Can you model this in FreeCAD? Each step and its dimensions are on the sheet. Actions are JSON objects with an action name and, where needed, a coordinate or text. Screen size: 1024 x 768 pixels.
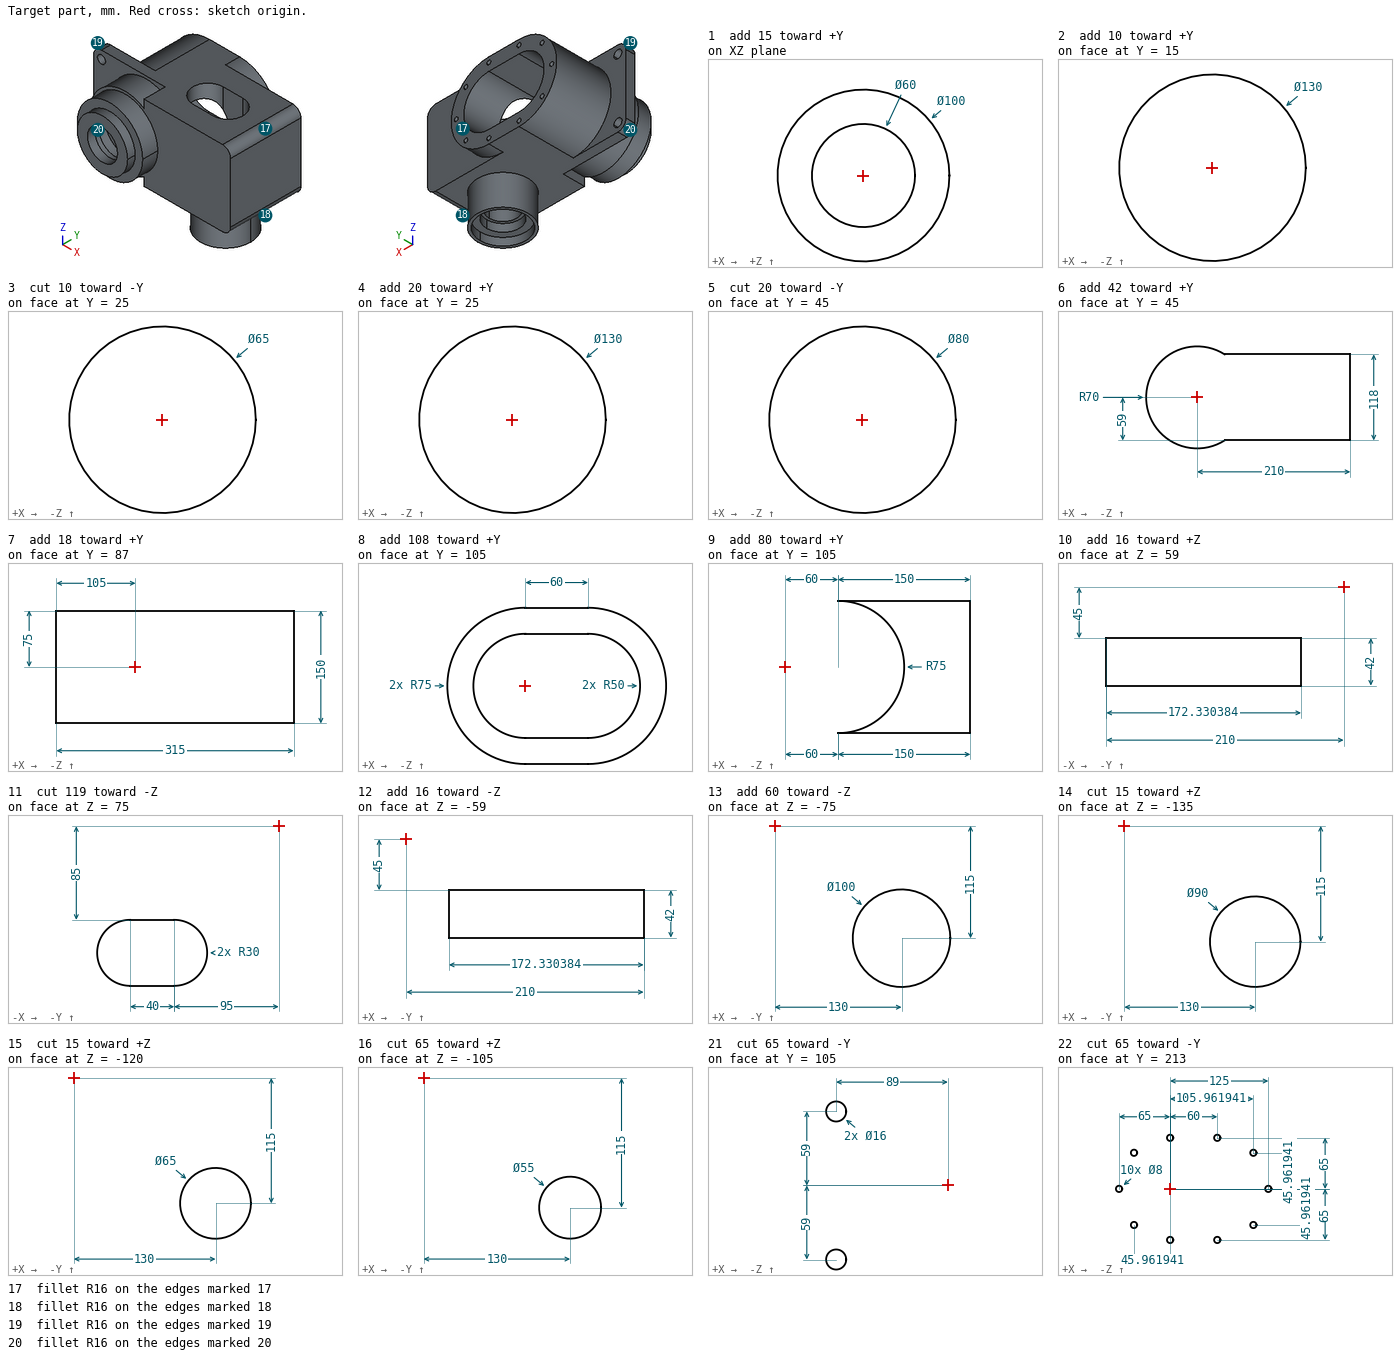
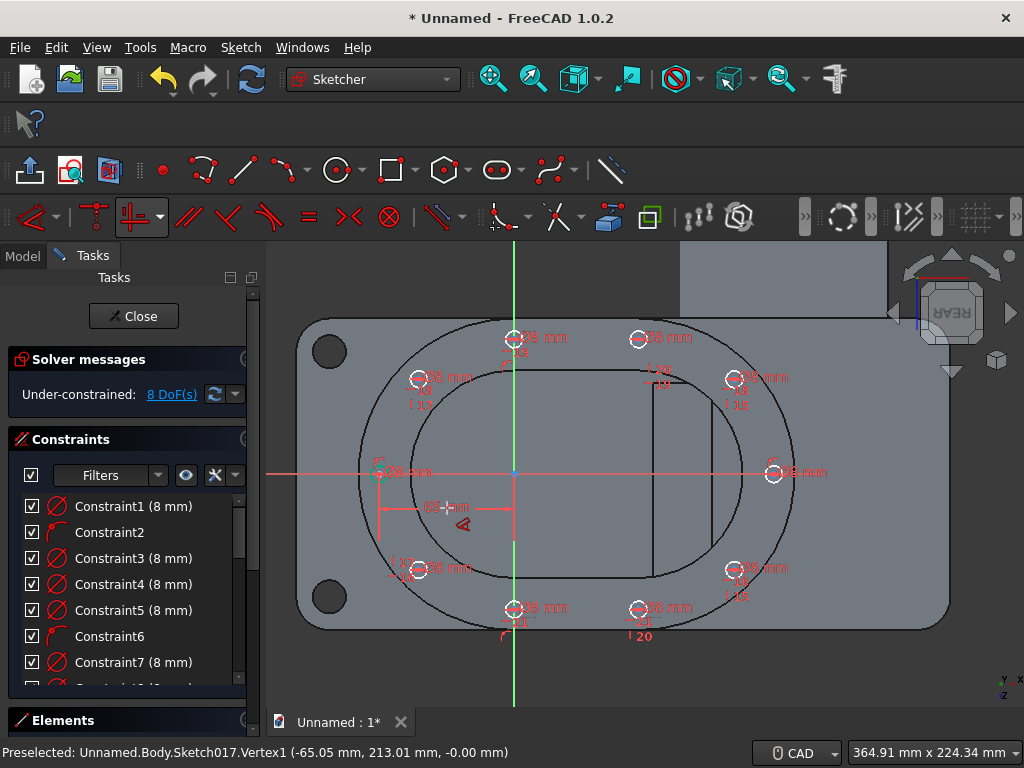
{"action": "left_click", "coordinate": [639, 339]}
{"action": "left_click", "coordinate": [576, 305]}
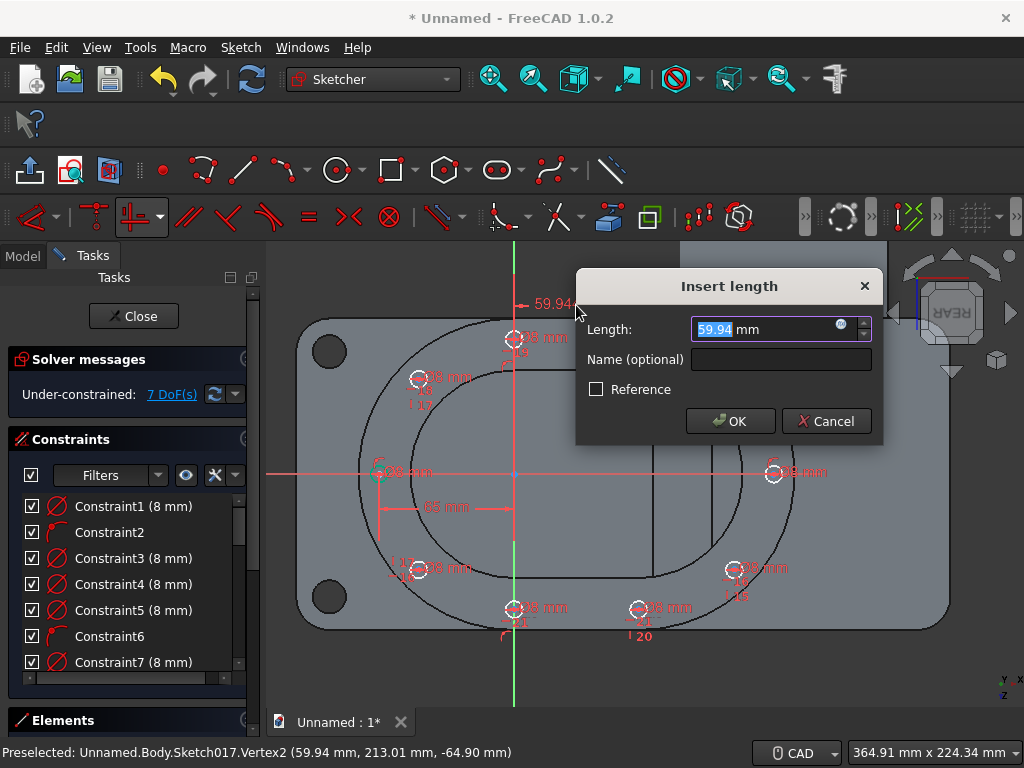
{"action": "type", "text": "60"}
{"action": "key", "text": "Return"}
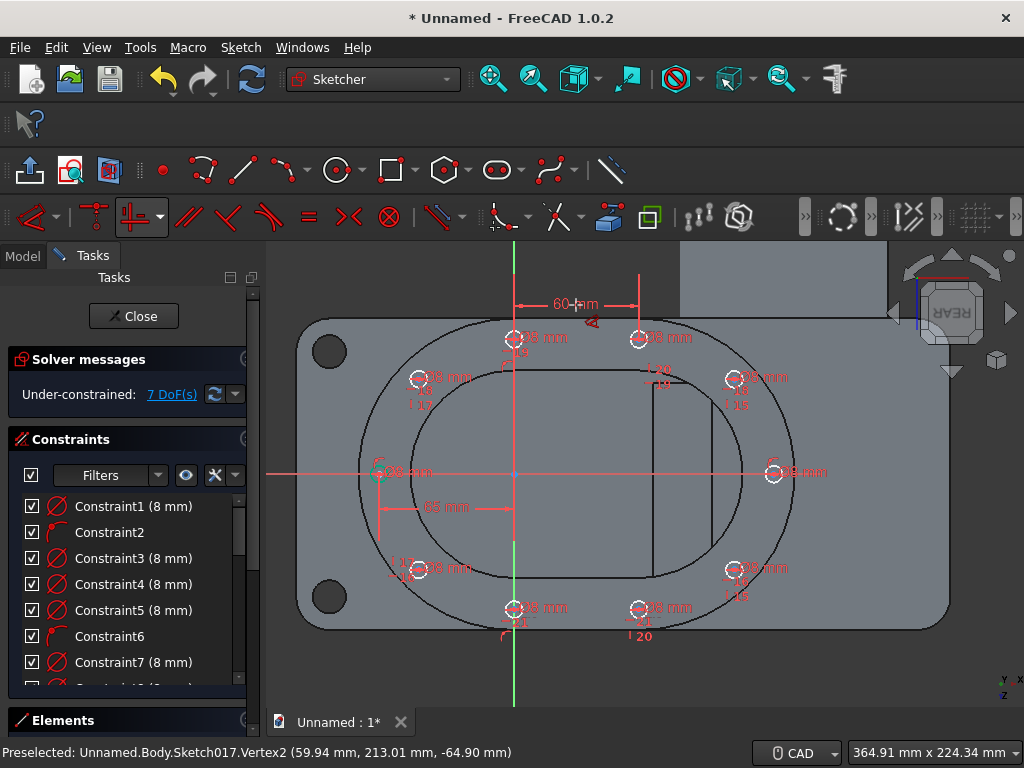
{"action": "left_click", "coordinate": [639, 339]}
{"action": "left_click", "coordinate": [673, 407]}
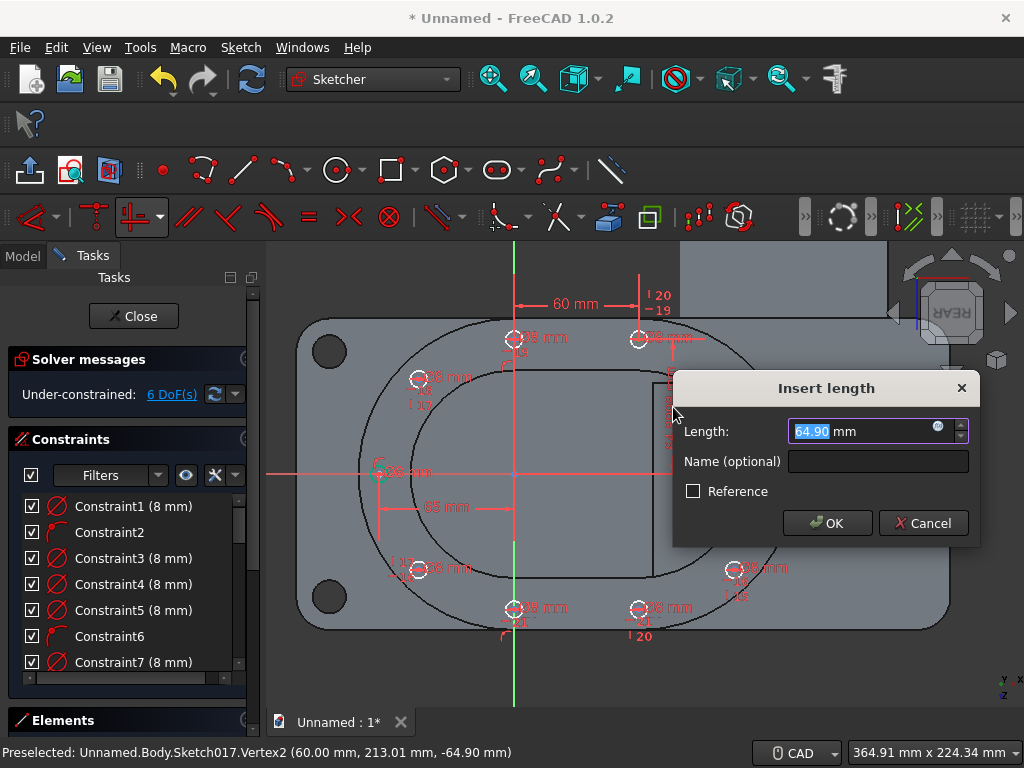
{"action": "type", "text": "65"}
{"action": "key", "text": "Return"}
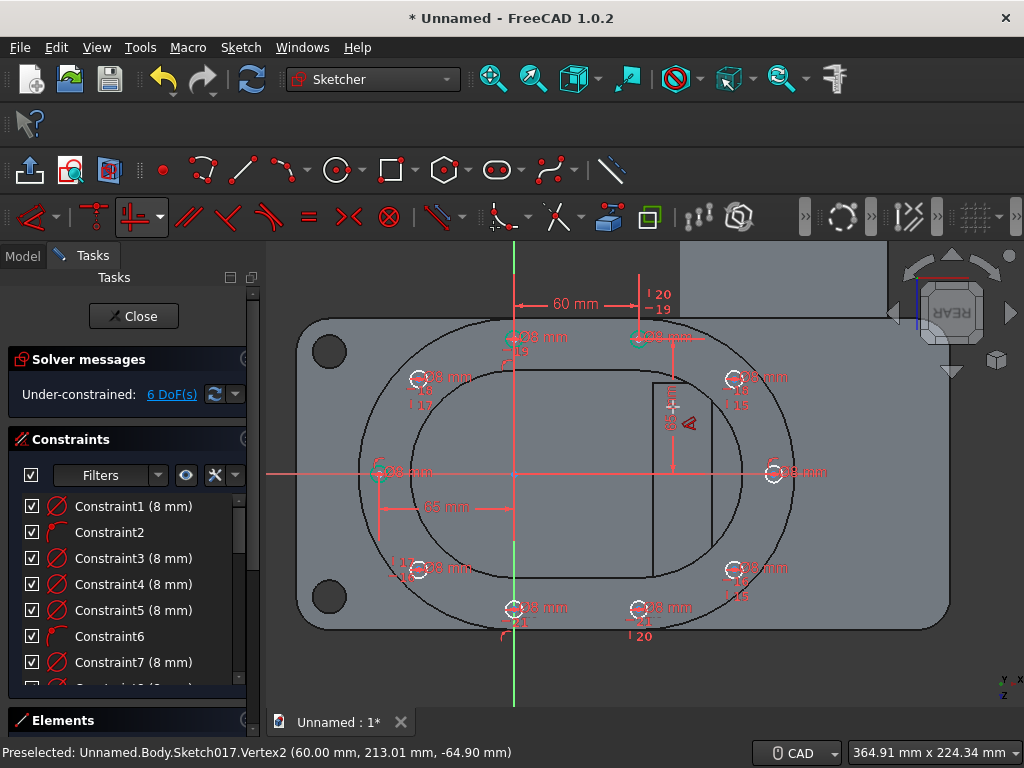
{"action": "left_click", "coordinate": [639, 610]}
{"action": "left_click", "coordinate": [673, 542]}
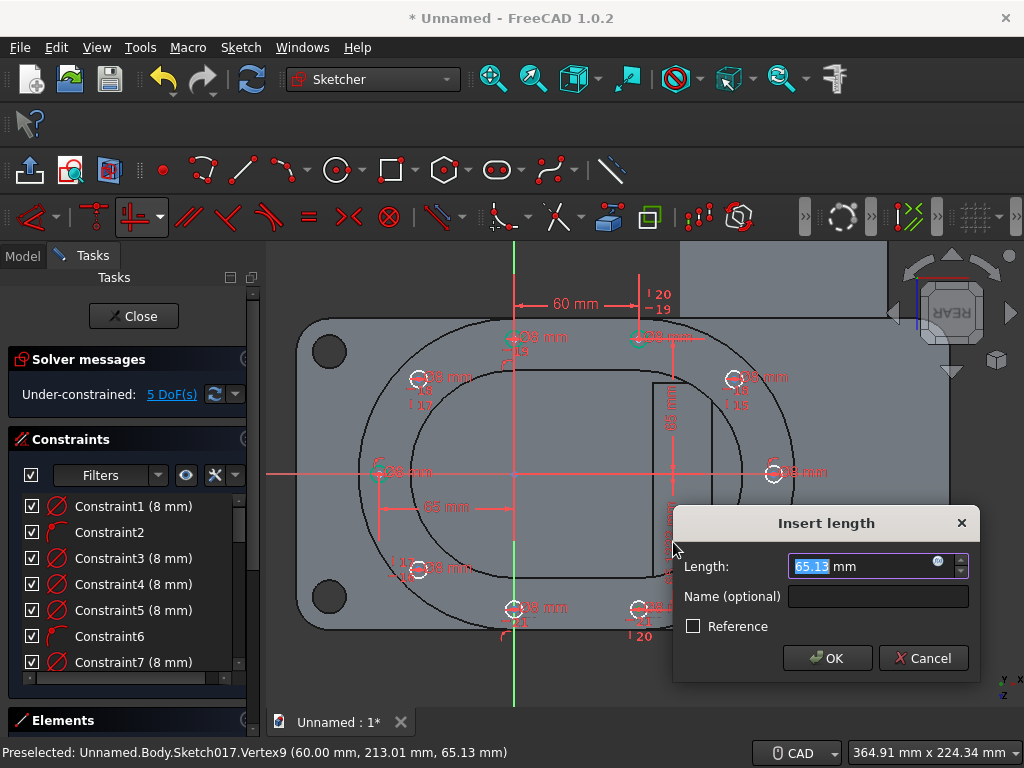
{"action": "type", "text": "65"}
{"action": "key", "text": "Return"}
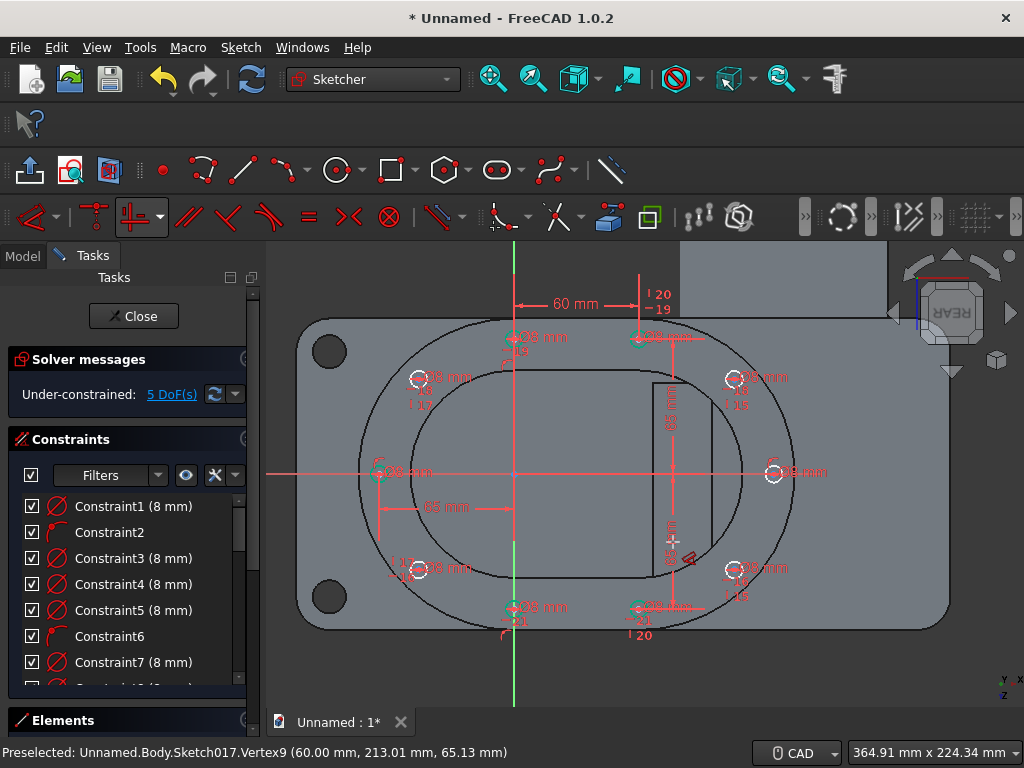
{"action": "left_click", "coordinate": [774, 474]}
{"action": "left_click", "coordinate": [644, 508]}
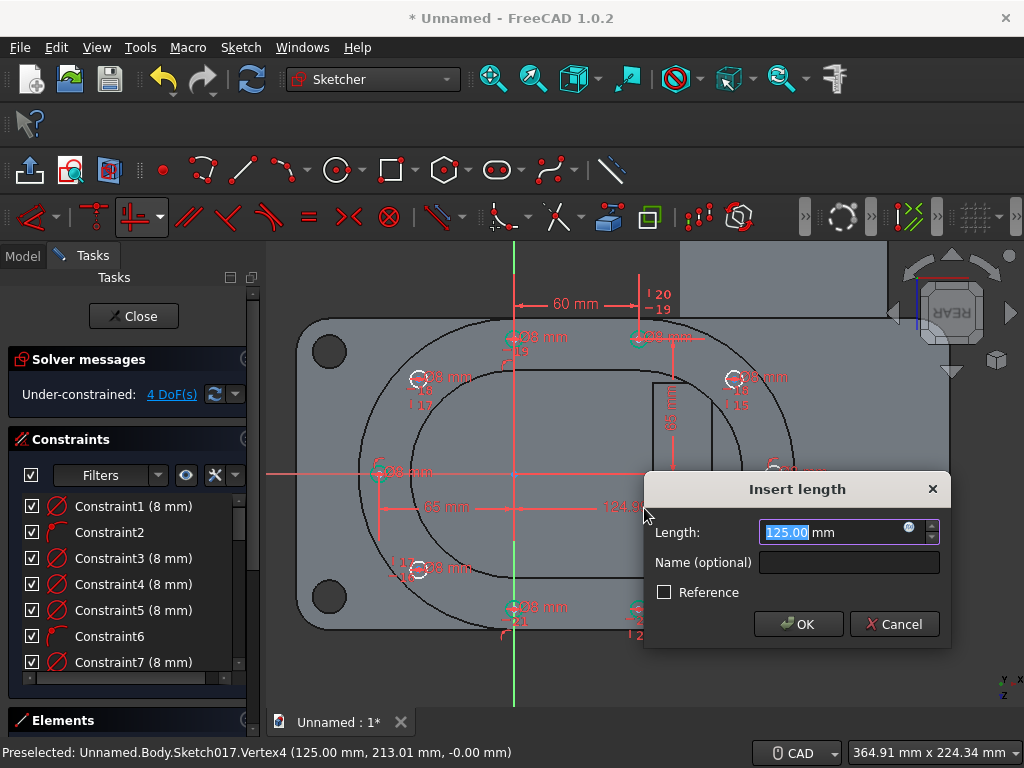
{"action": "type", "text": "125"}
{"action": "key", "text": "Return"}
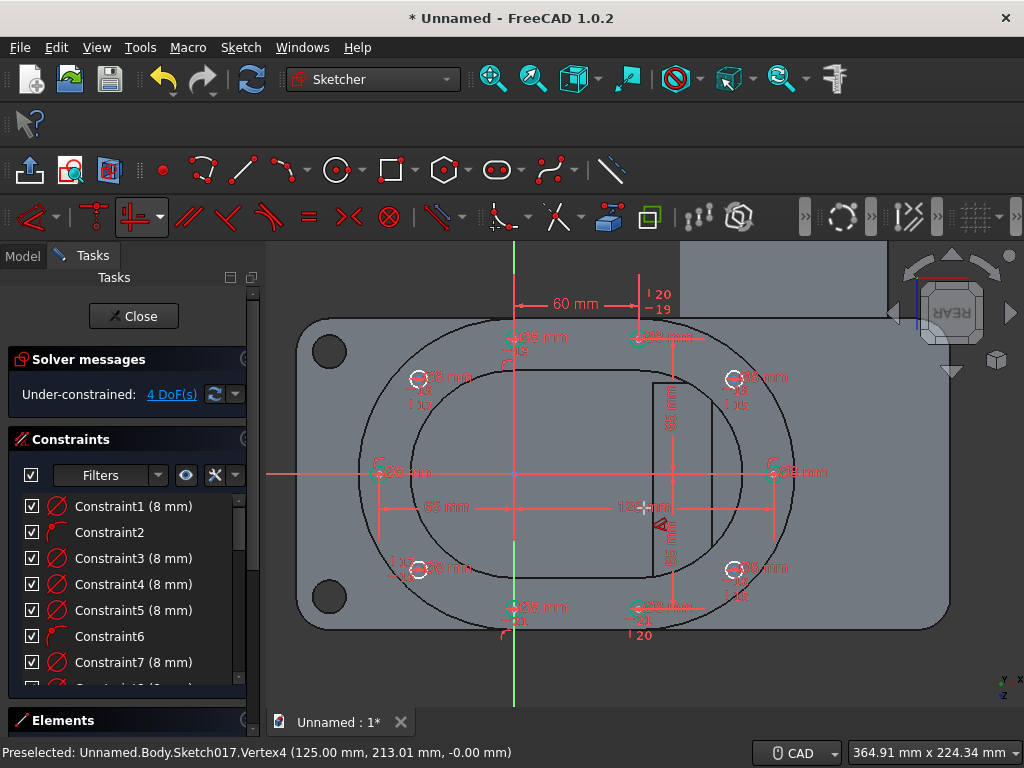
{"action": "left_click", "coordinate": [734, 379]}
{"action": "left_click", "coordinate": [768, 427]}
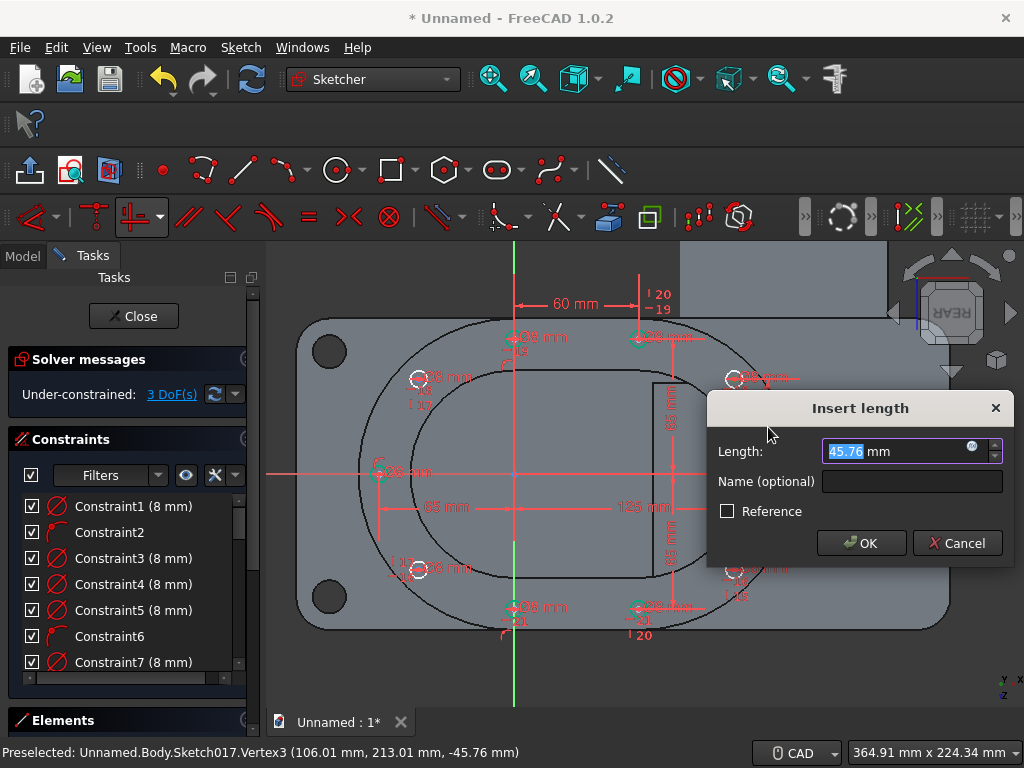
{"action": "type", "text": "45.961941"}
{"action": "key", "text": "Return"}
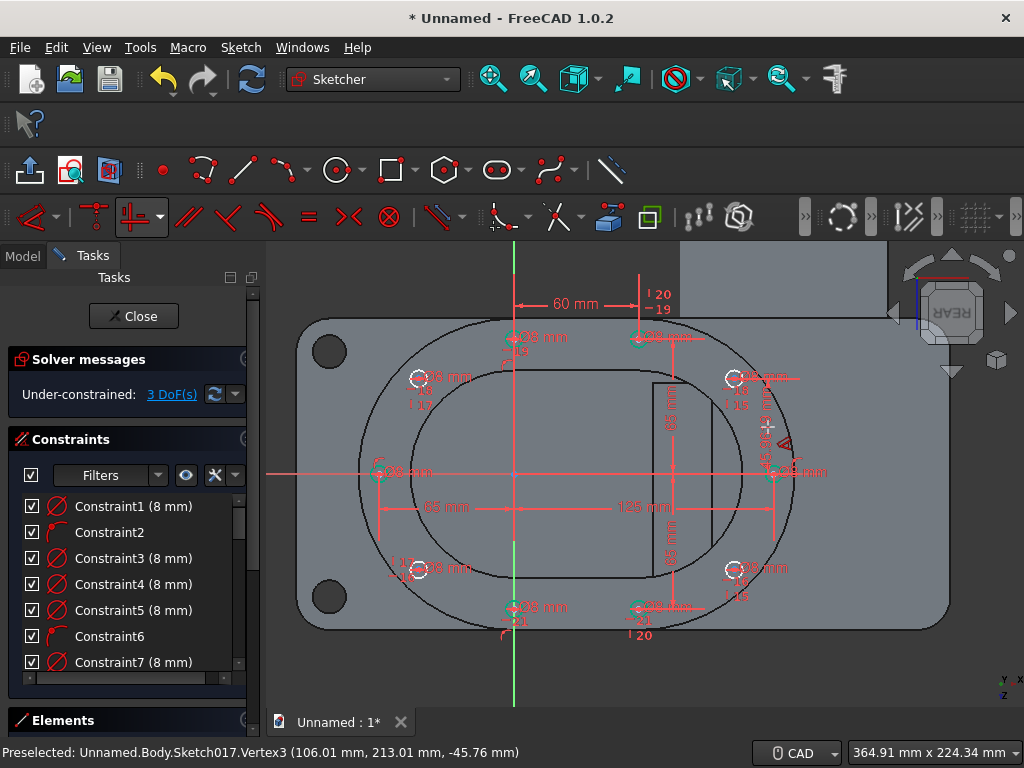
{"action": "left_click", "coordinate": [734, 570]}
{"action": "left_click", "coordinate": [768, 522]}